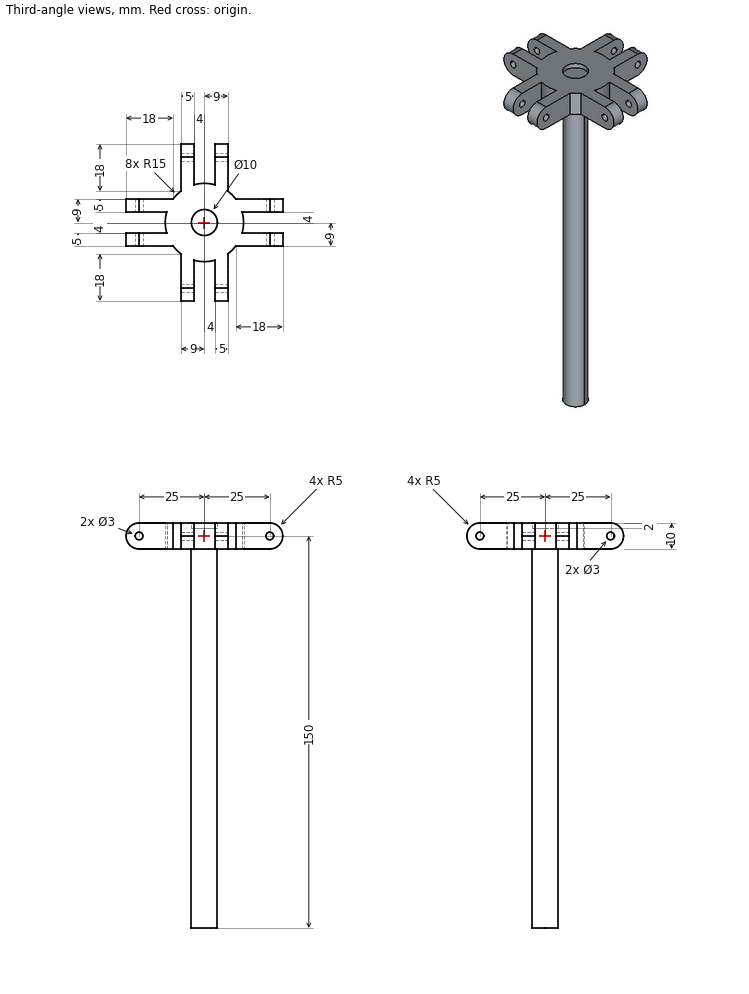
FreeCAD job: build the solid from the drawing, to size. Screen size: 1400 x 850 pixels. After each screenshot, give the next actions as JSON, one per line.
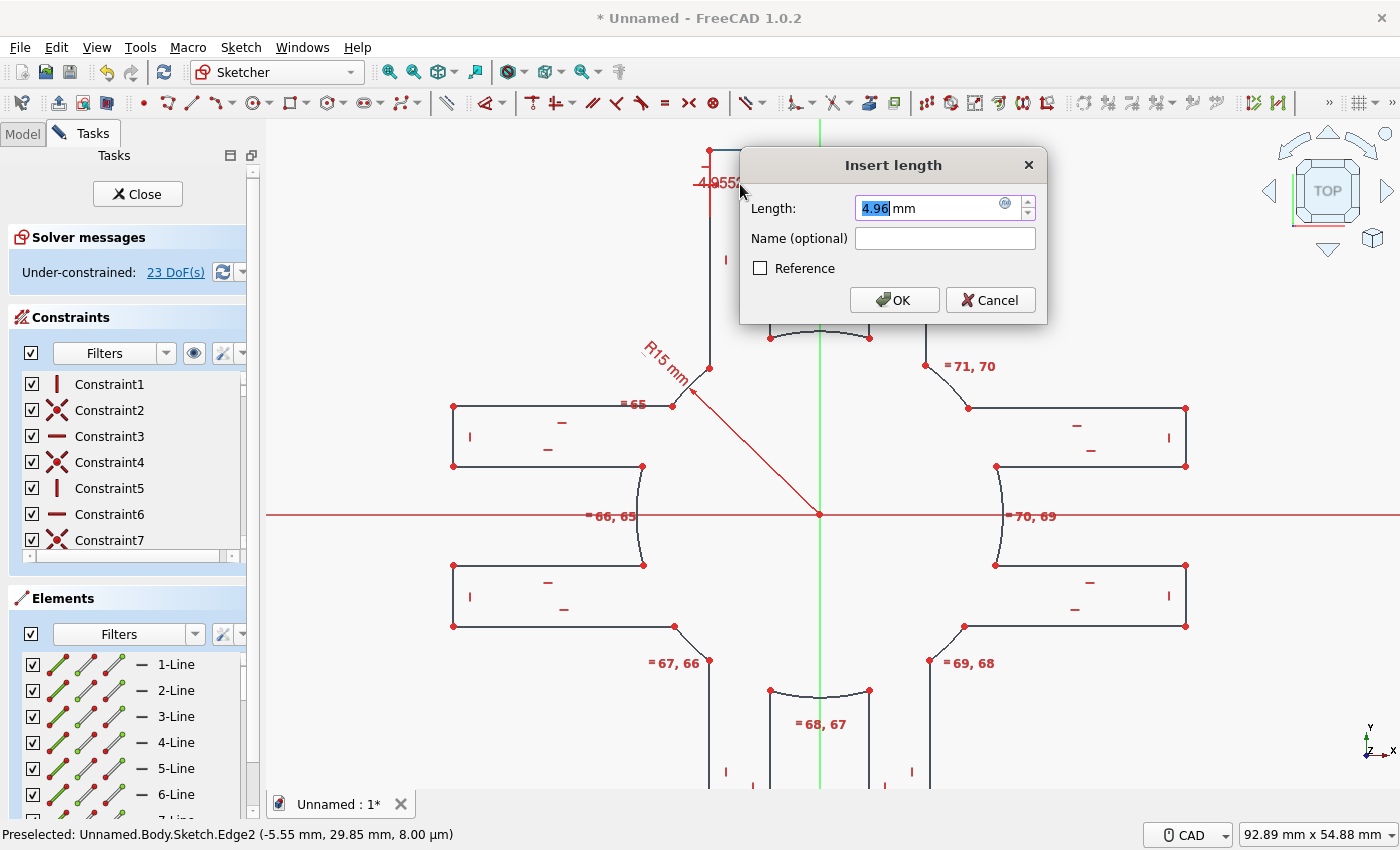
{"action": "type", "text": "5"}
{"action": "key", "text": "Return"}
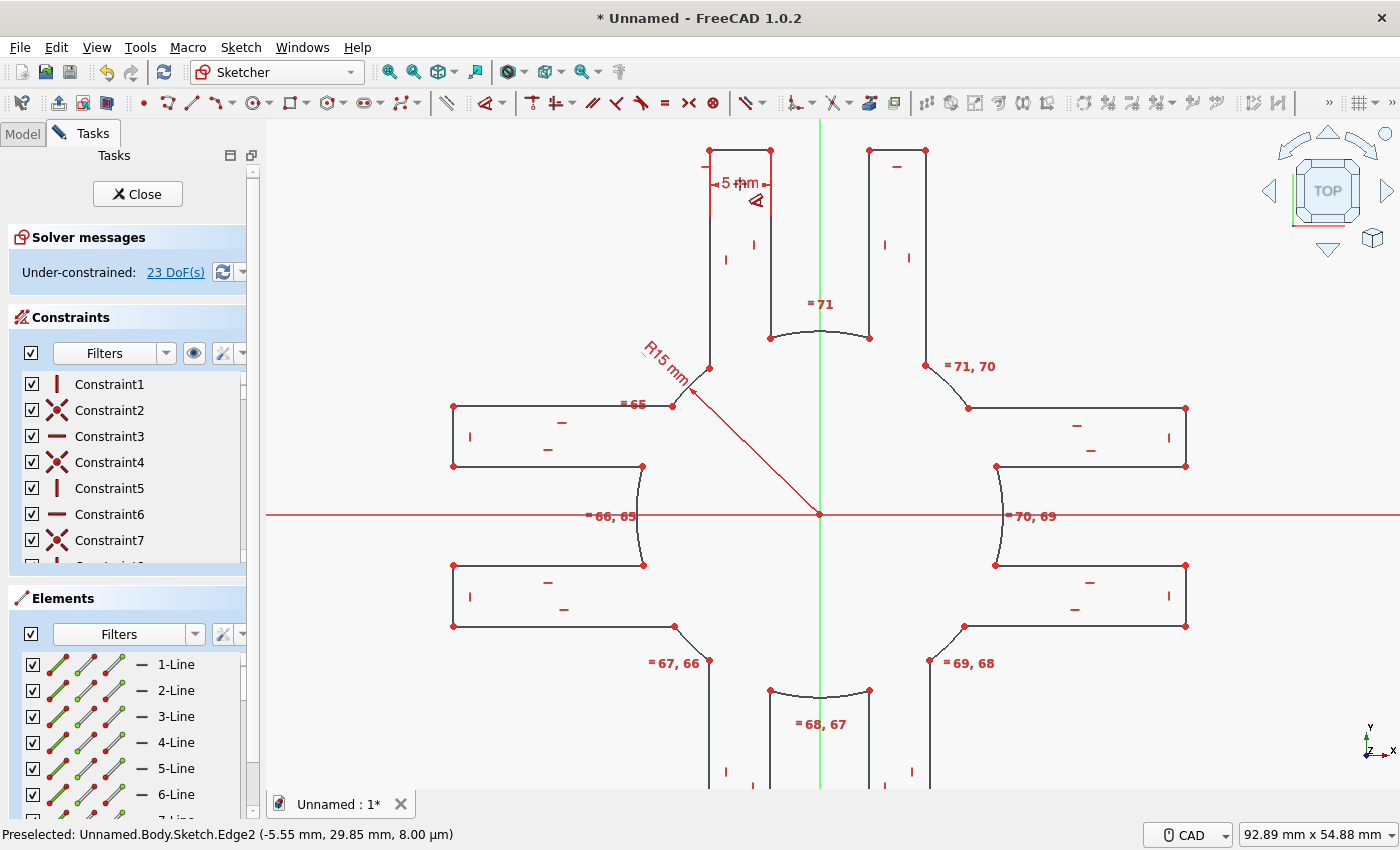
{"action": "left_click", "coordinate": [453, 424]}
{"action": "left_click", "coordinate": [419, 436]}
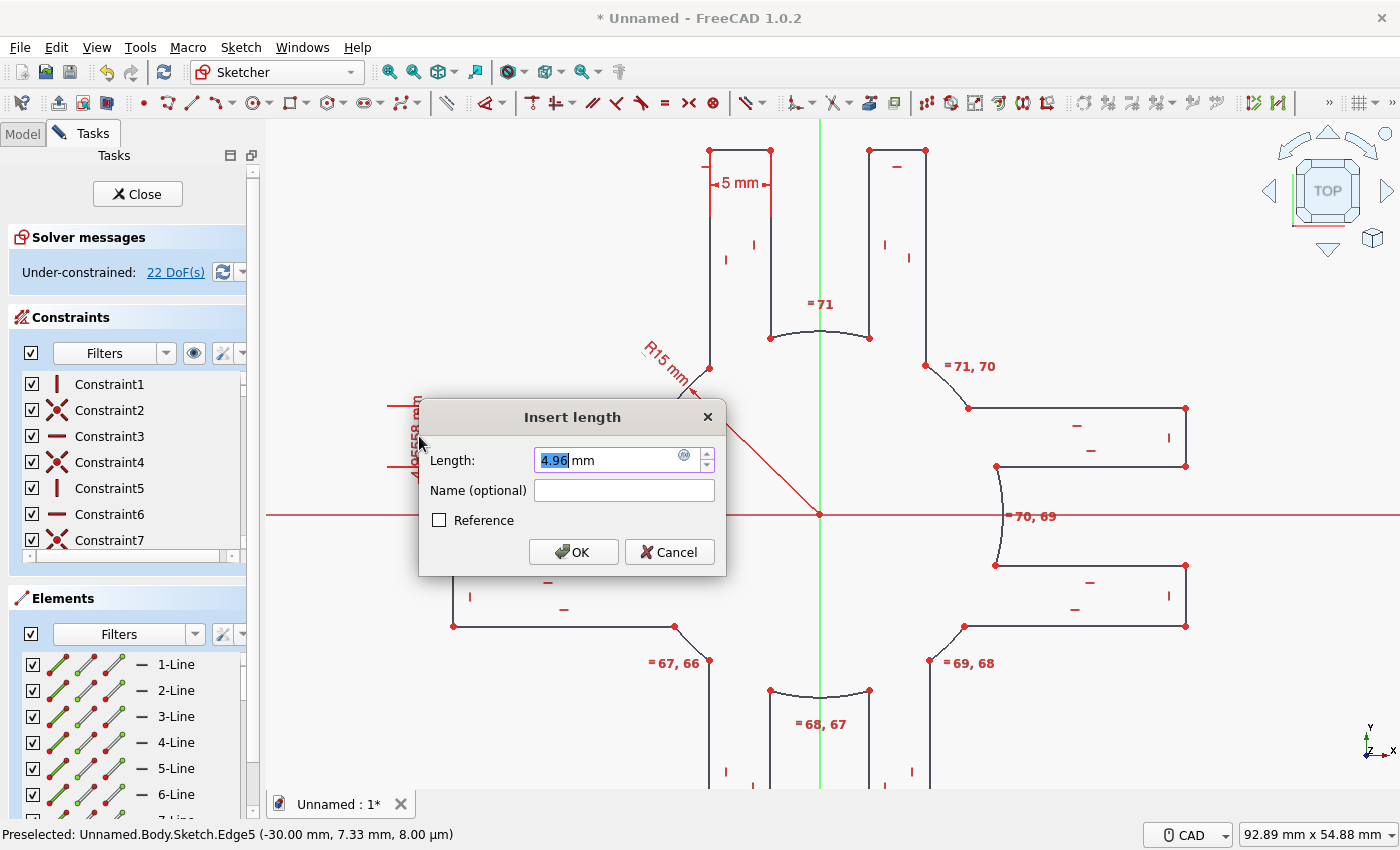
{"action": "type", "text": "5"}
{"action": "key", "text": "Return"}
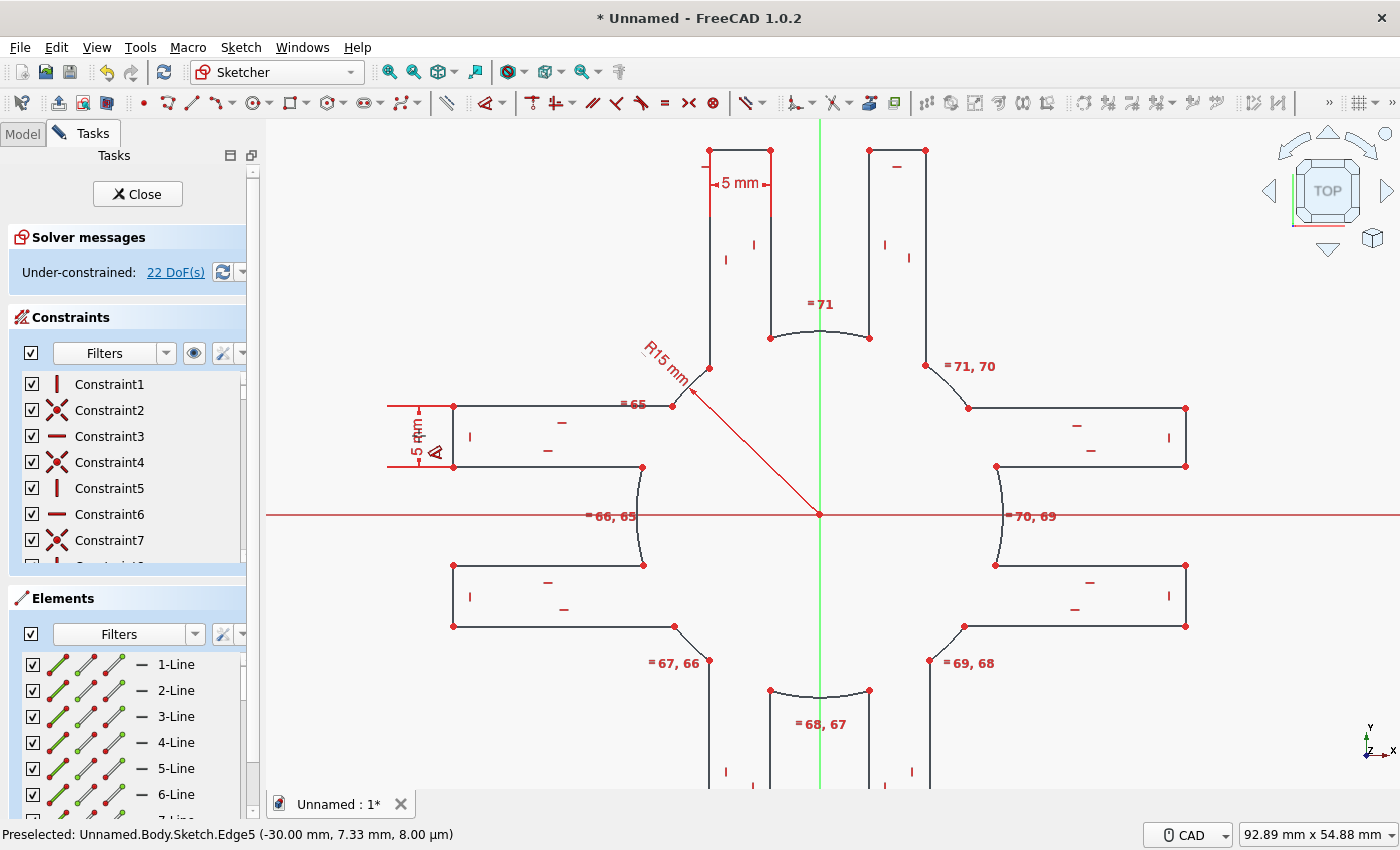
{"action": "left_click", "coordinate": [453, 584]}
{"action": "left_click", "coordinate": [419, 596]}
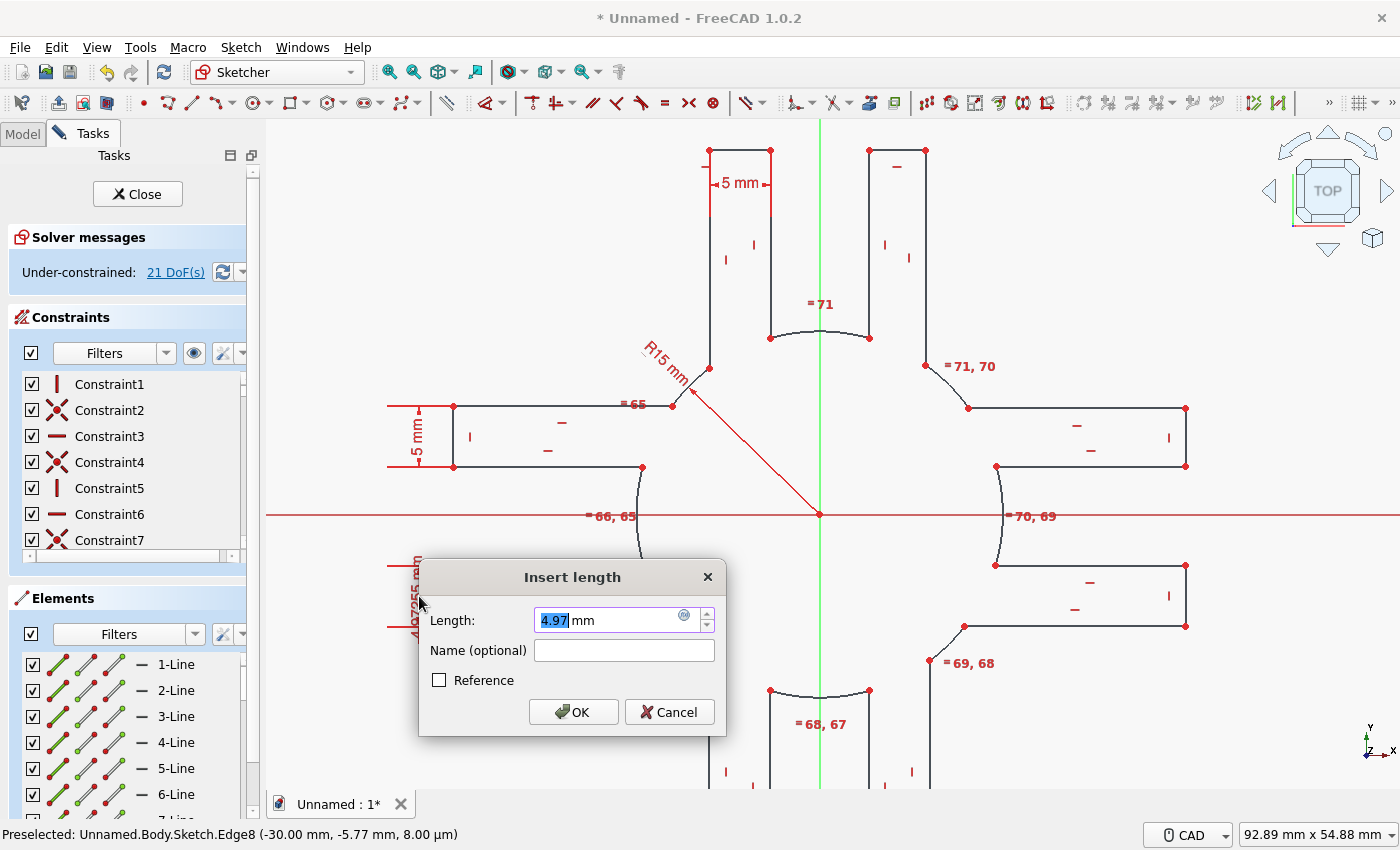
{"action": "type", "text": "5"}
{"action": "key", "text": "Return"}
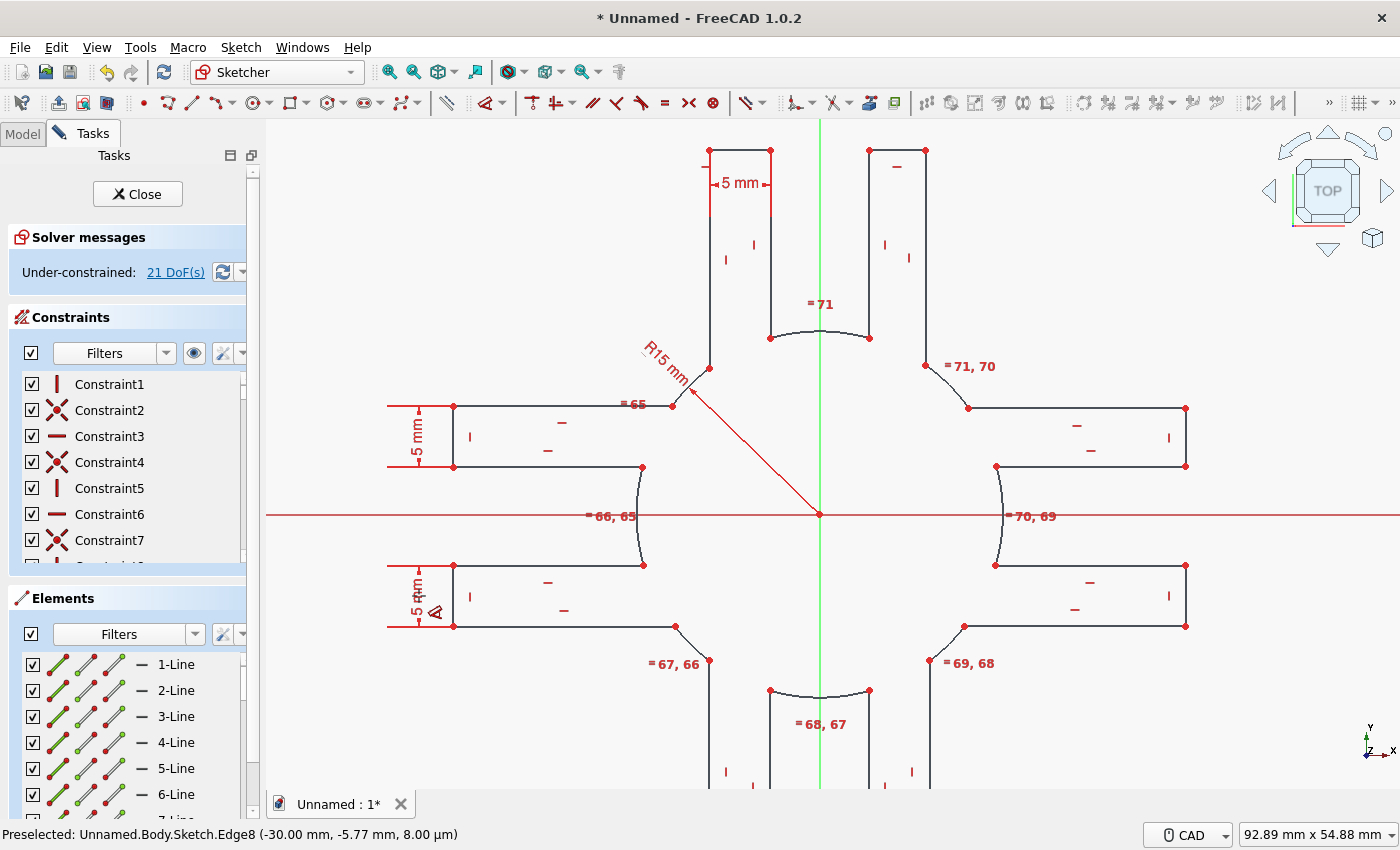
{"action": "scroll", "coordinate": [697, 380], "scroll_direction": "down", "scroll_amount": 3}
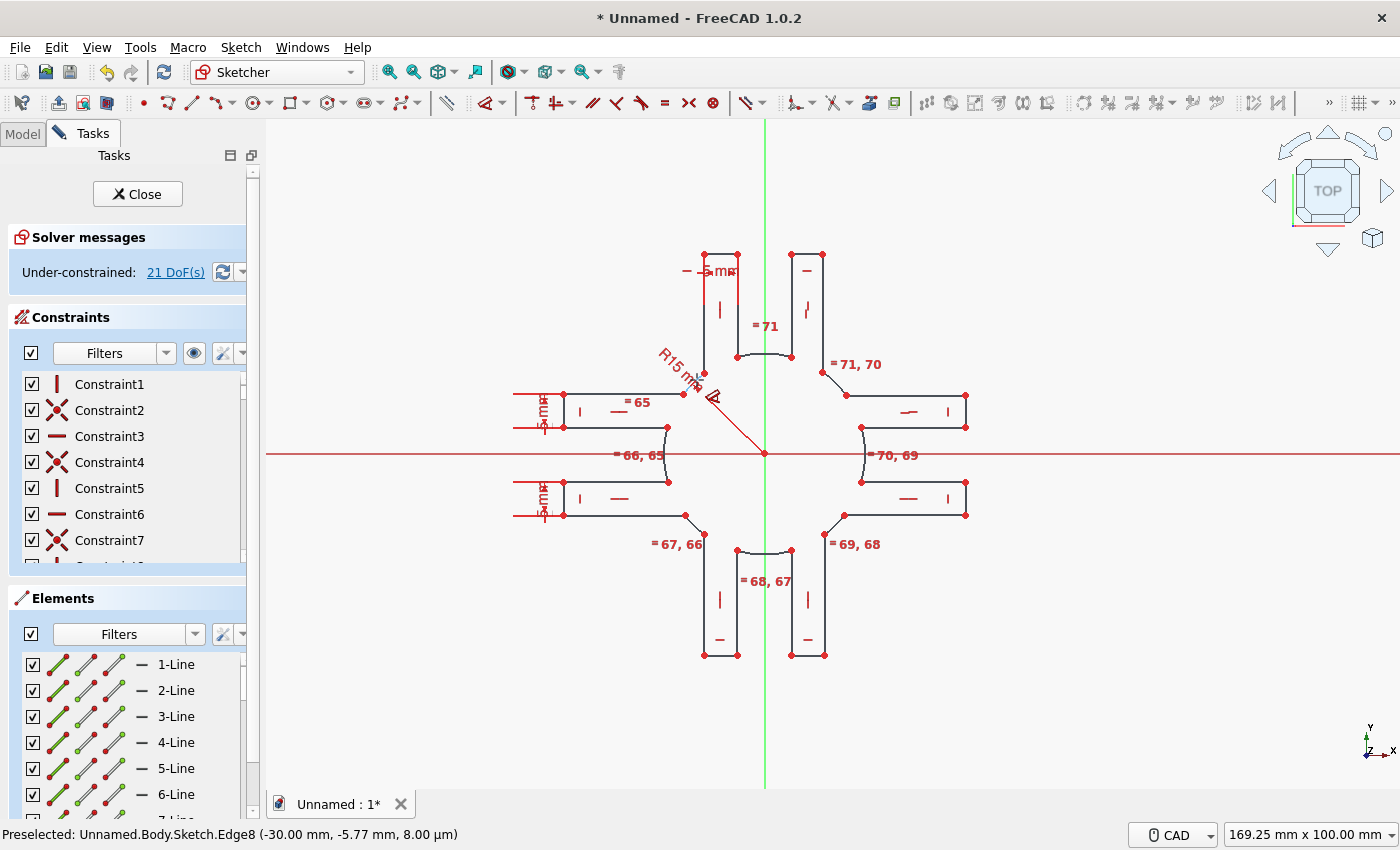
{"action": "scroll", "coordinate": [714, 656], "scroll_direction": "up", "scroll_amount": 2}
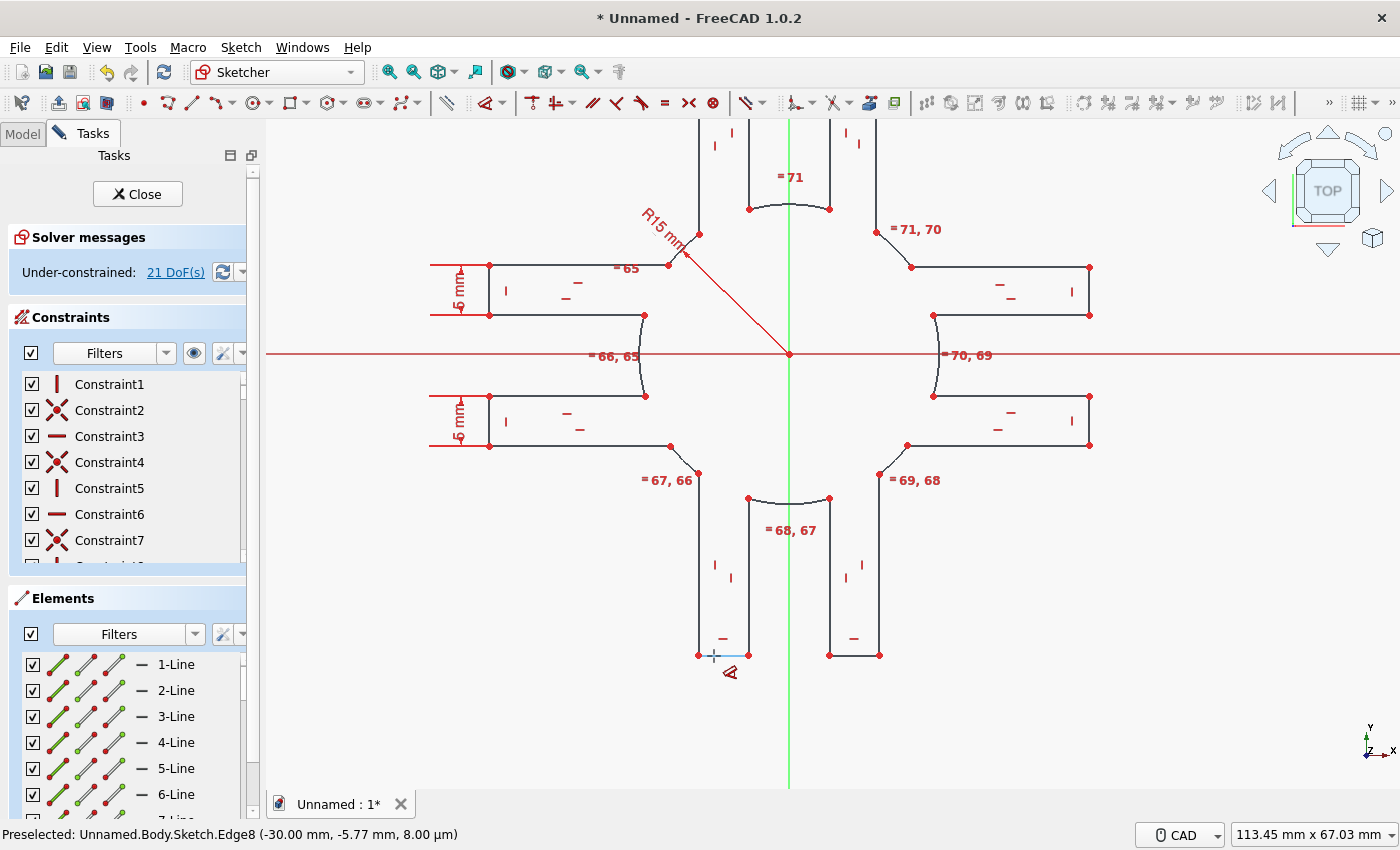
{"action": "left_click", "coordinate": [714, 656]}
{"action": "left_click", "coordinate": [724, 690]}